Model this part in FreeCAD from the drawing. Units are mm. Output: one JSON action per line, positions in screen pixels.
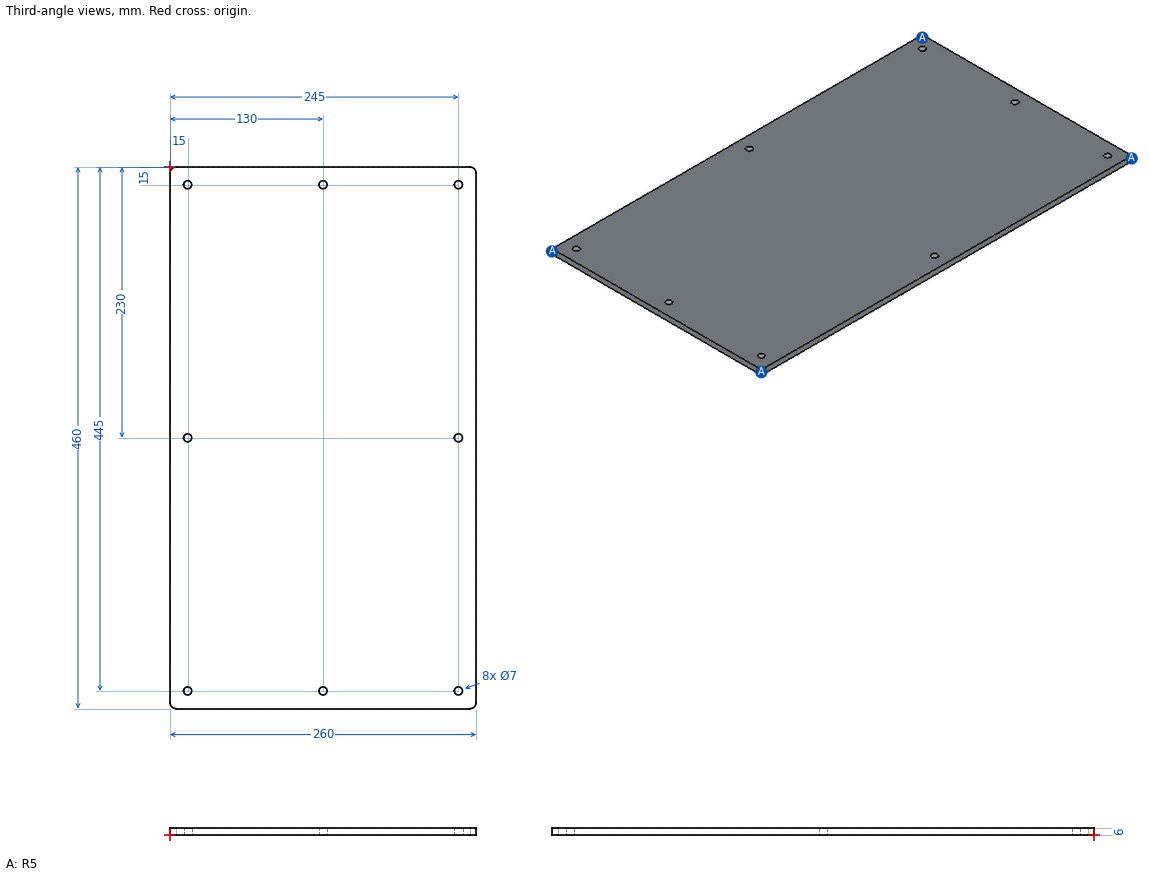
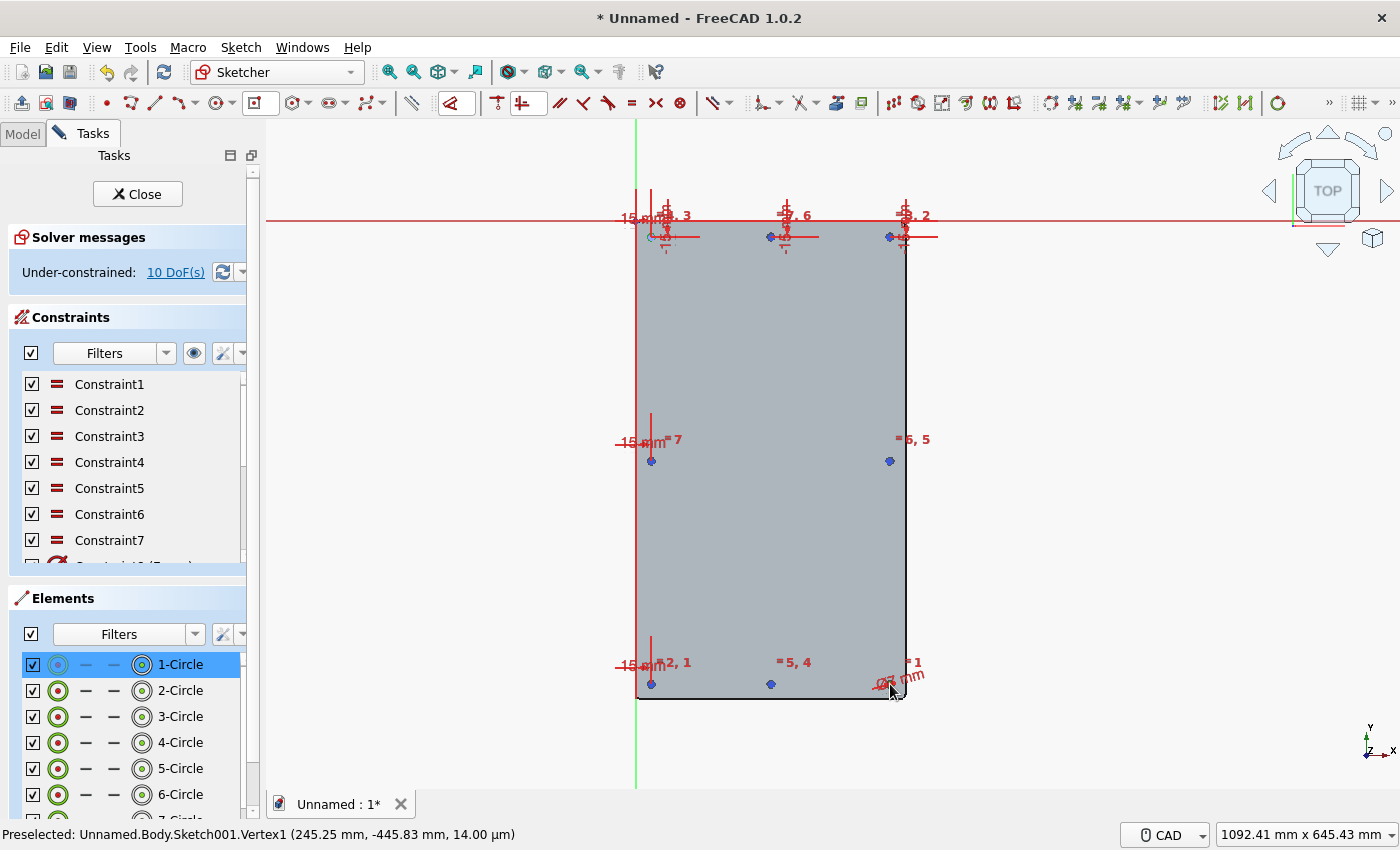
{"action": "key", "text": "l"}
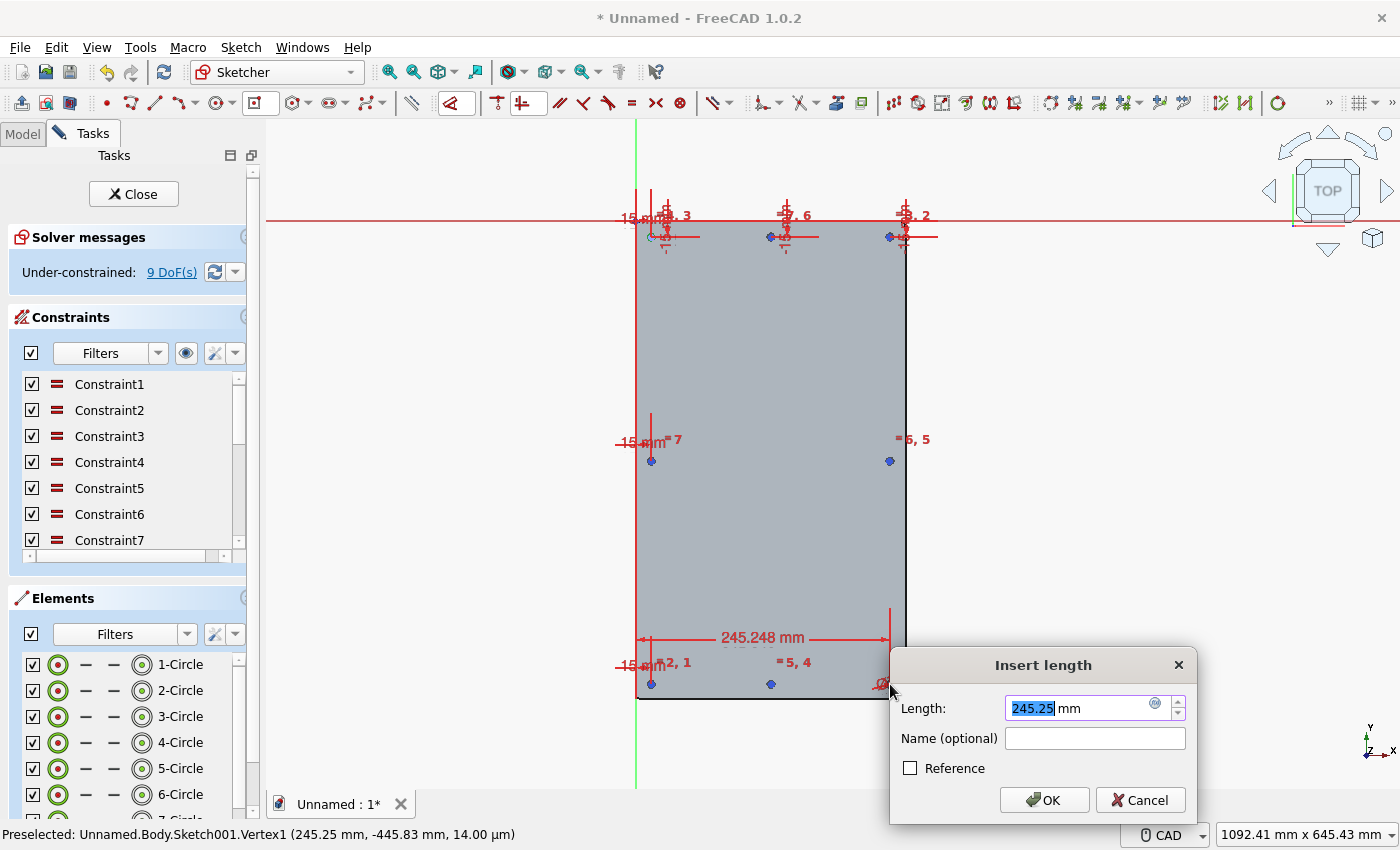
{"action": "type", "text": "245"}
{"action": "key", "text": "Return"}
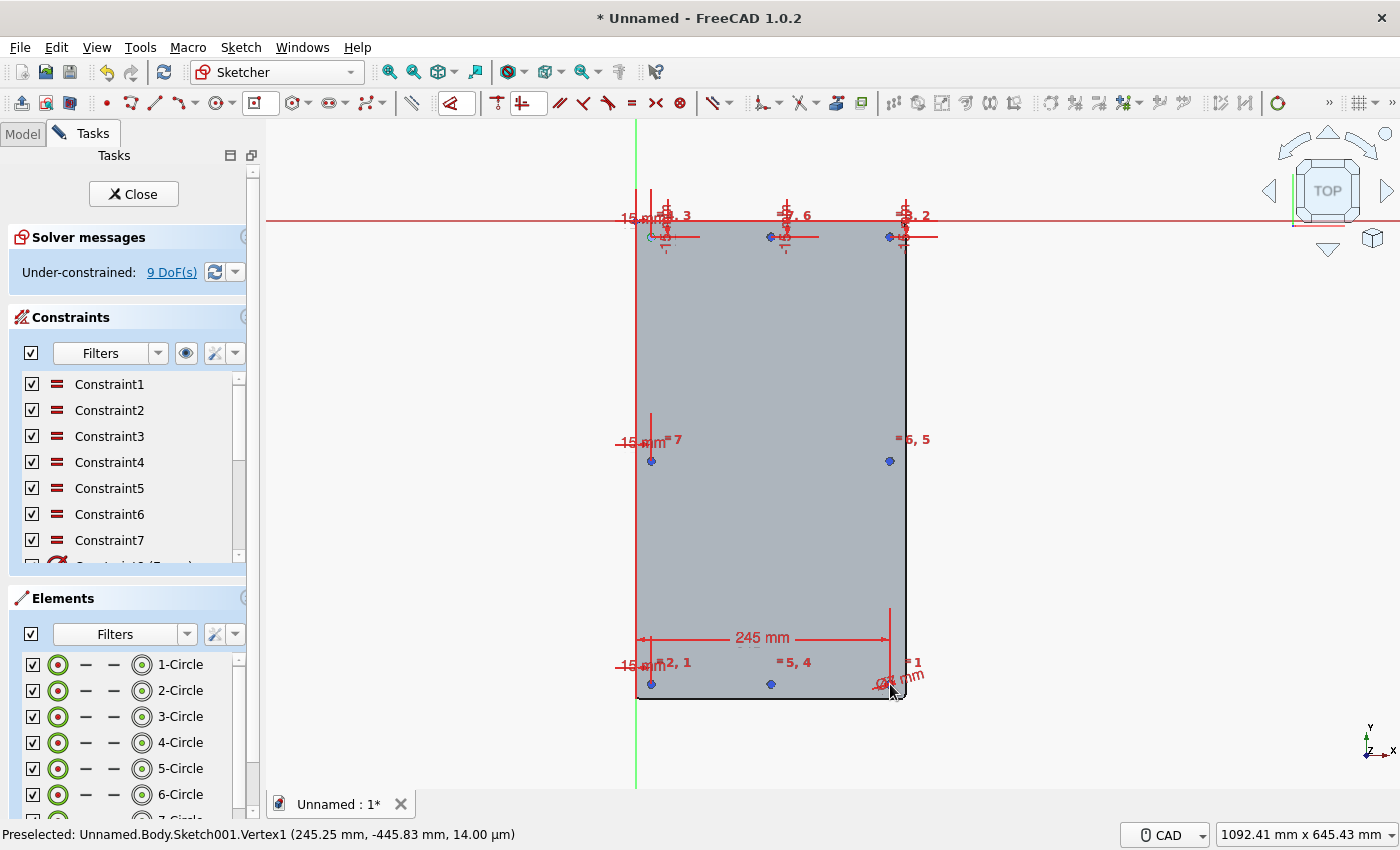
{"action": "left_click", "coordinate": [890, 684]}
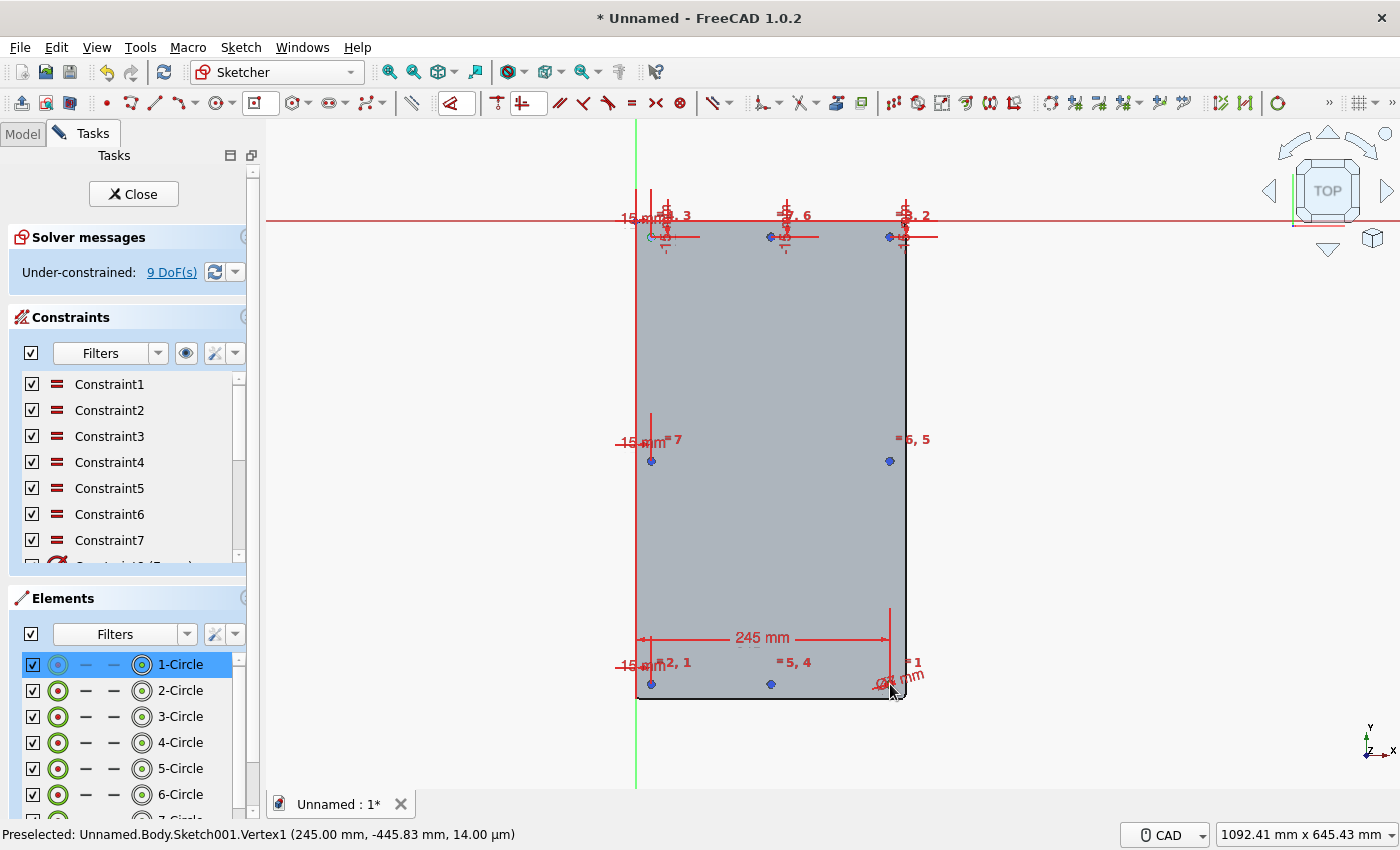
{"action": "key", "text": "i"}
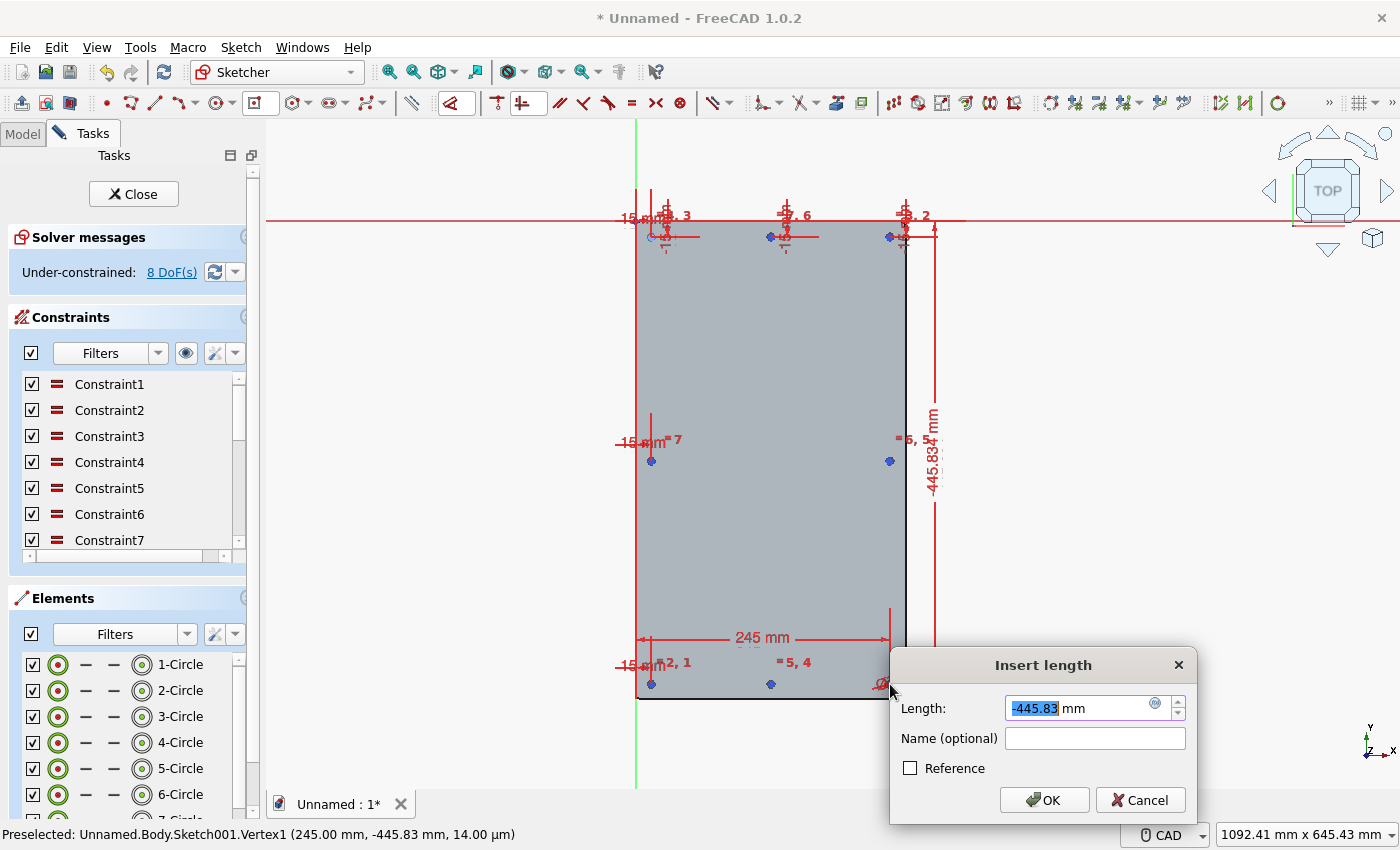
{"action": "type", "text": "-445"}
{"action": "key", "text": "Return"}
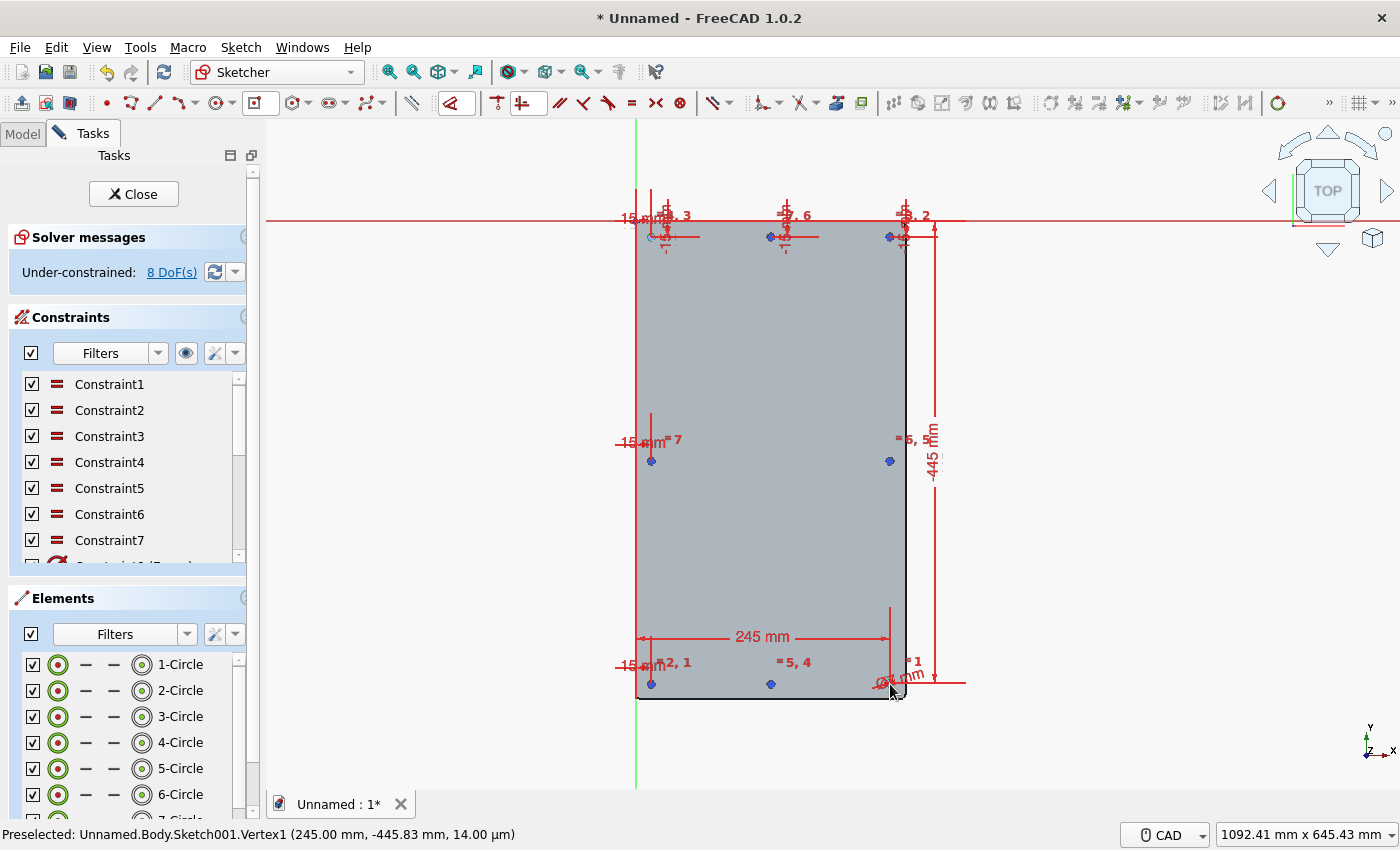
{"action": "left_click", "coordinate": [651, 684]}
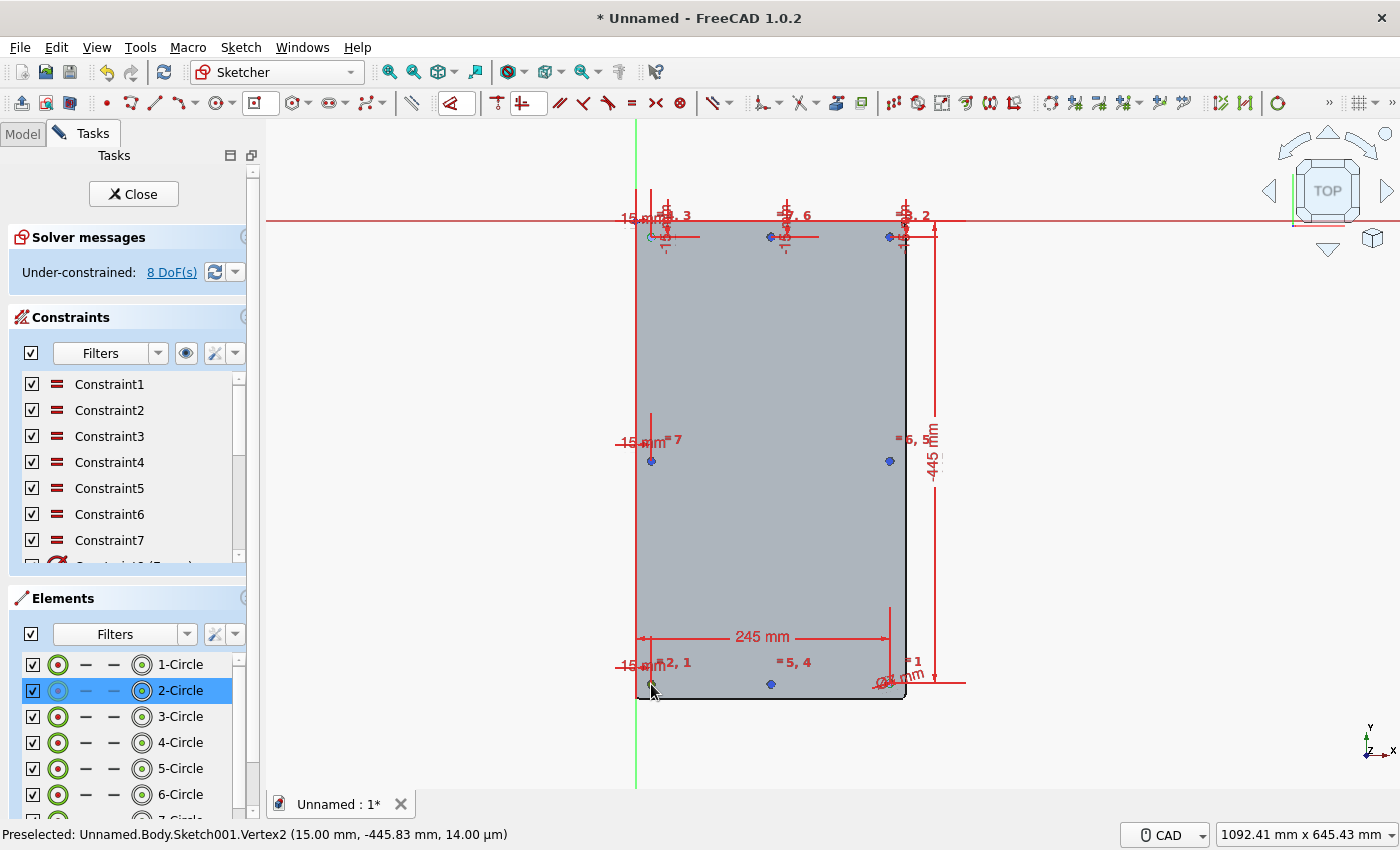
{"action": "key", "text": "i"}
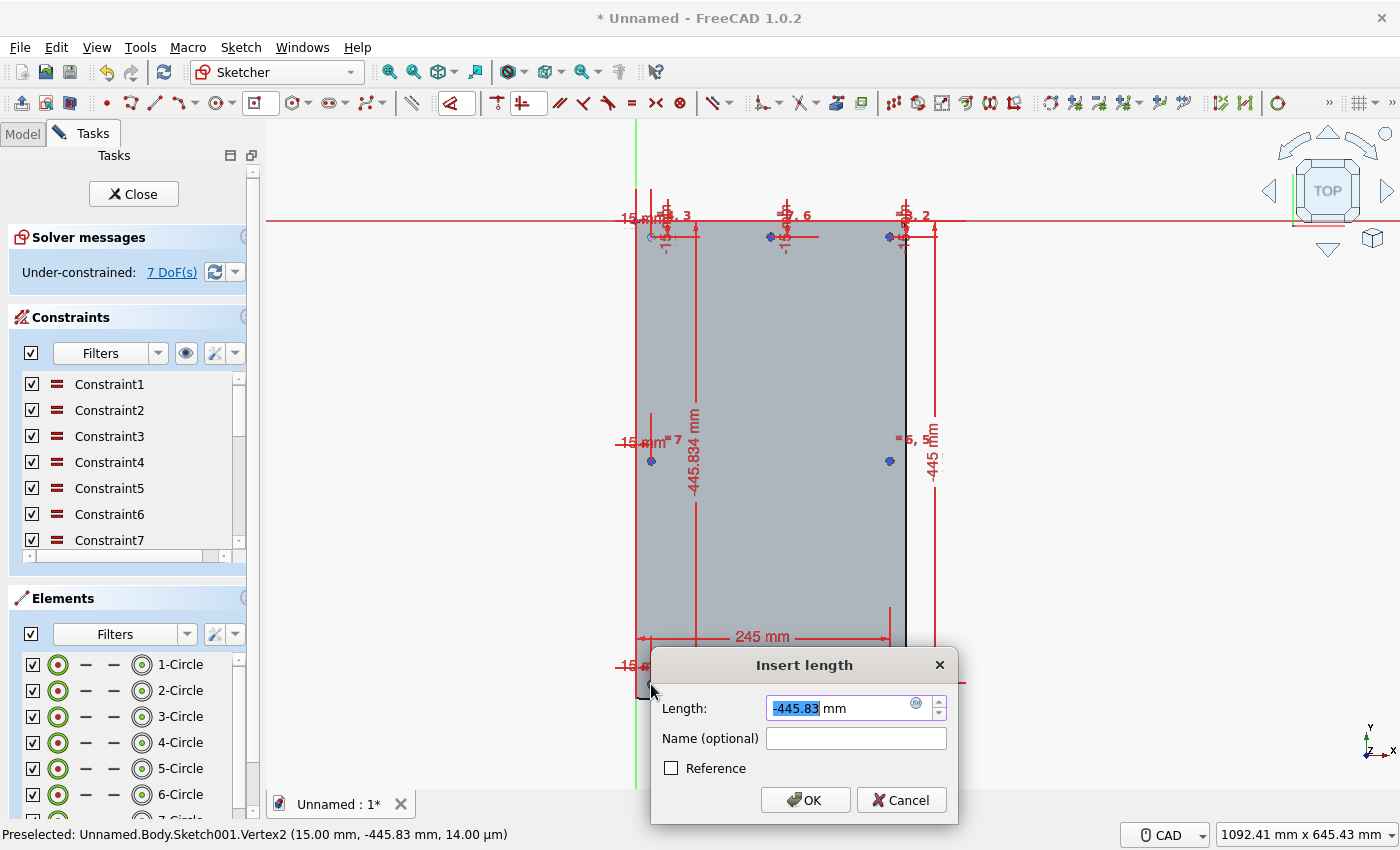
{"action": "type", "text": "-445"}
{"action": "key", "text": "Return"}